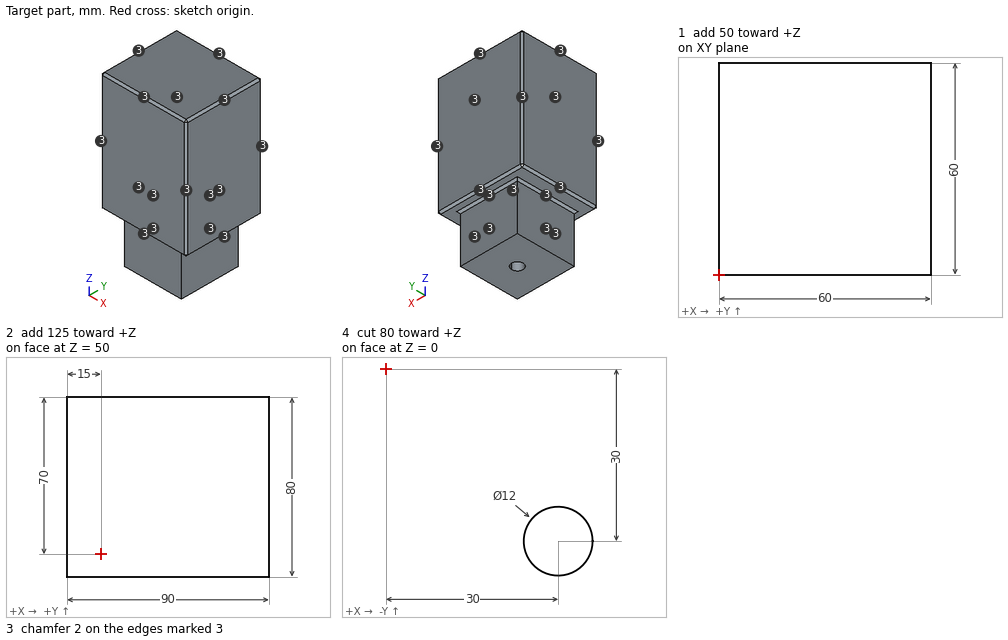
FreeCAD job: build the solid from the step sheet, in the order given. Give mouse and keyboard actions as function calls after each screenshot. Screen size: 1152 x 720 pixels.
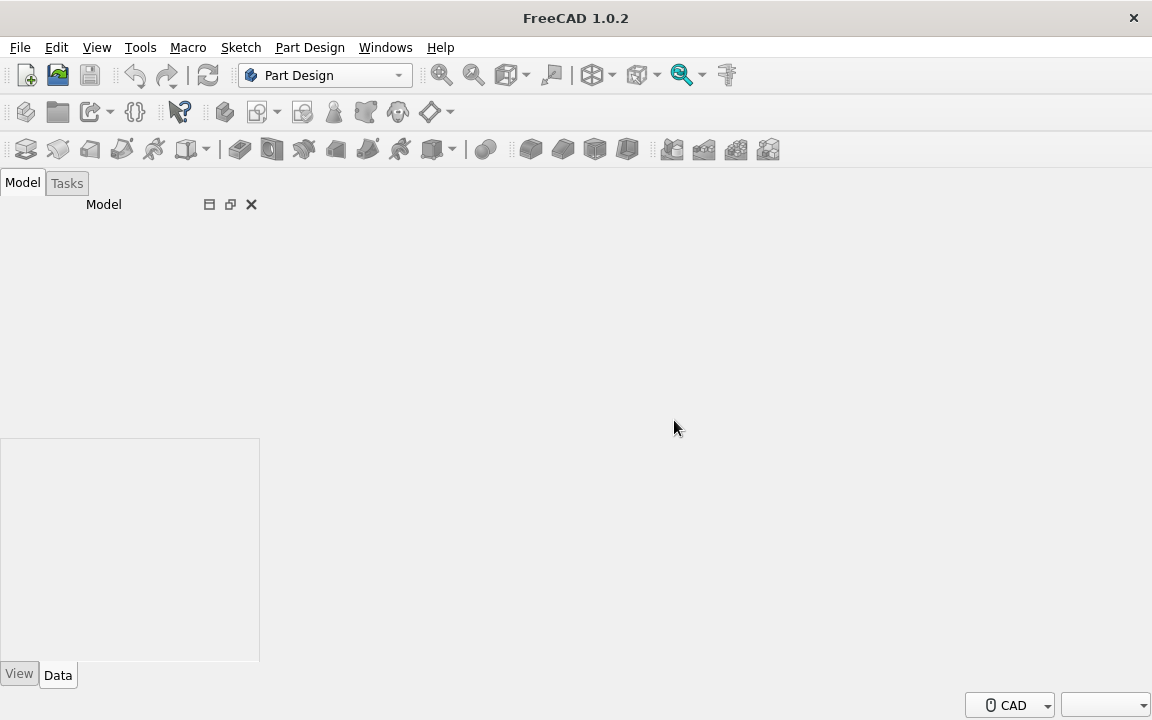
key(ctrl+n)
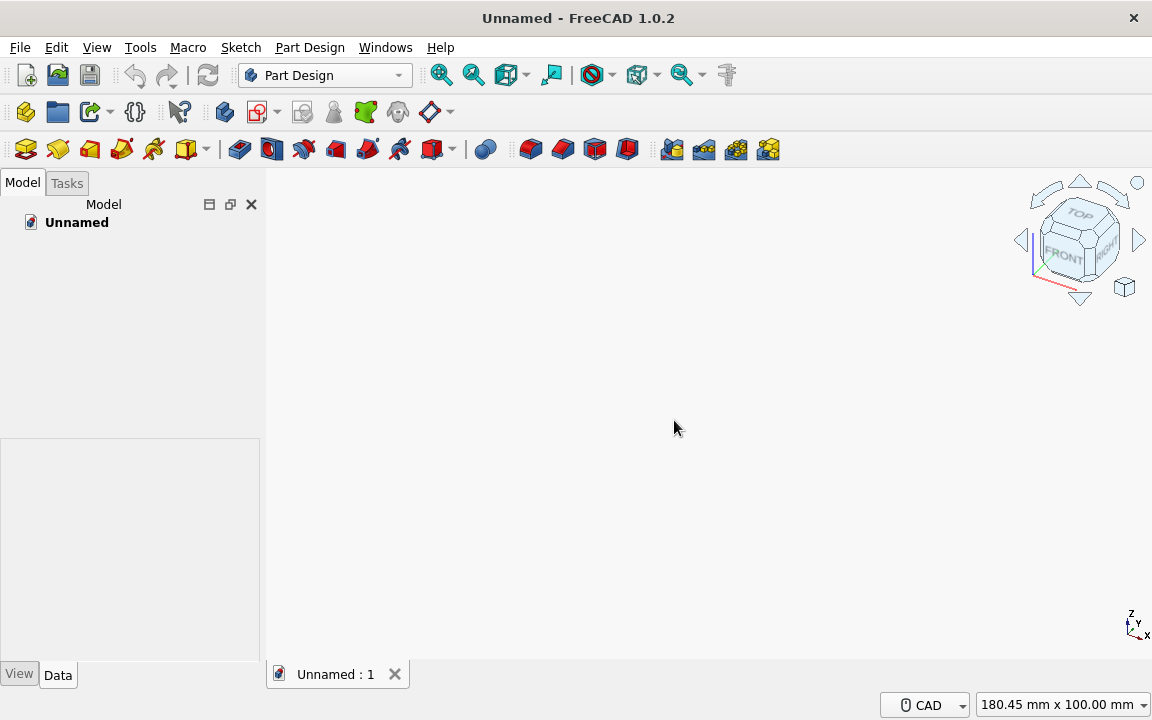
click(258, 112)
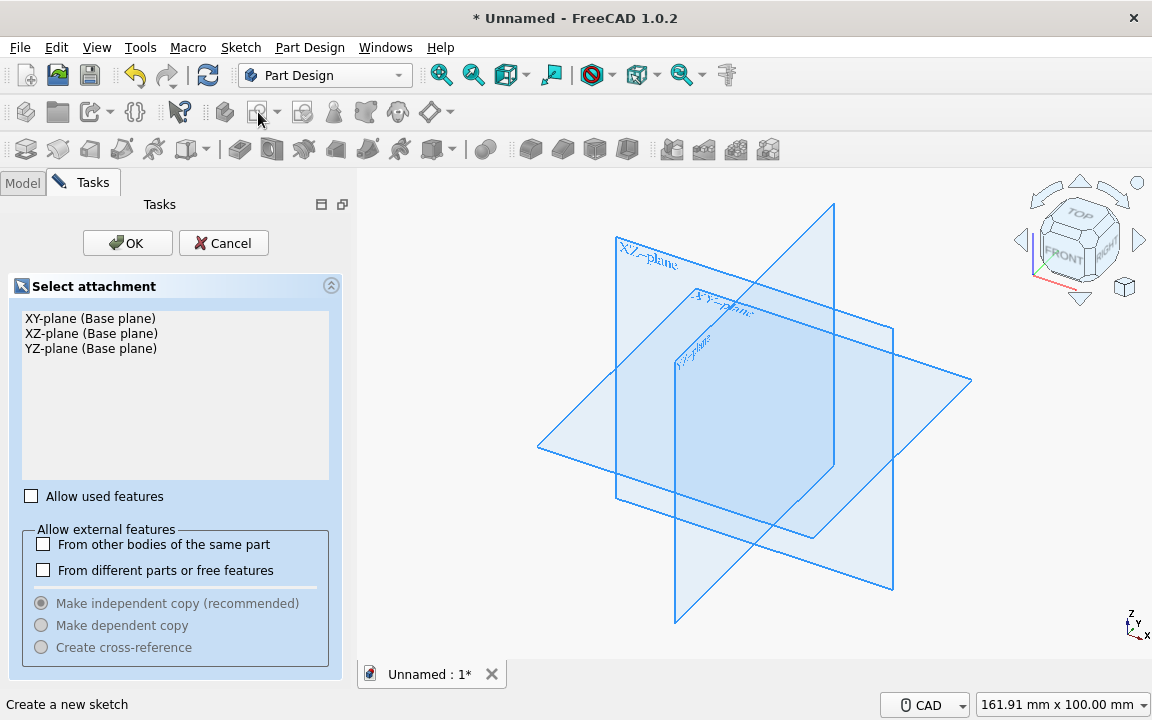
click(82, 318)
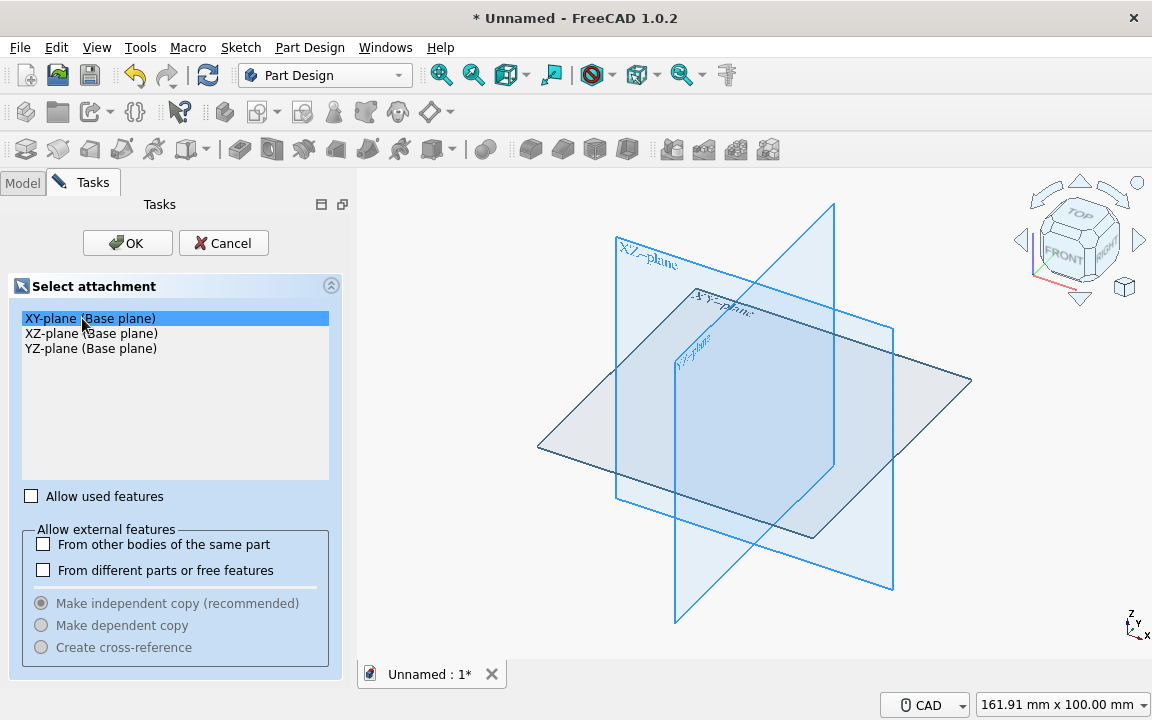
click(128, 243)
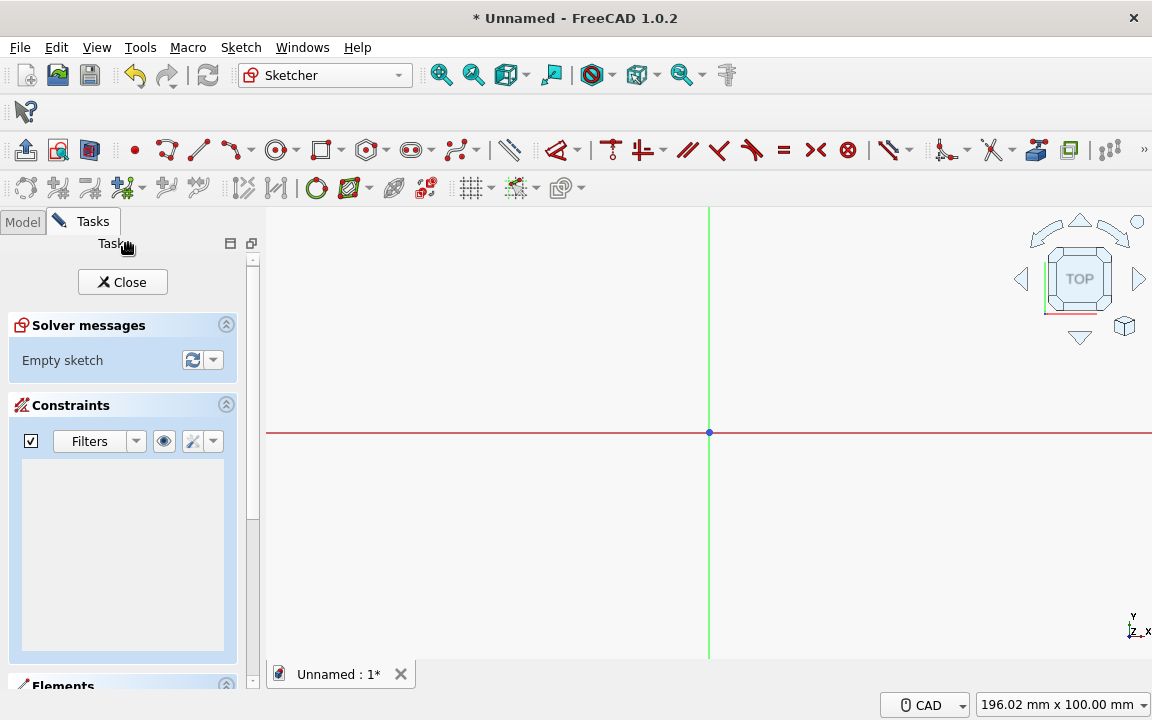
scroll(294, 631, down, 2)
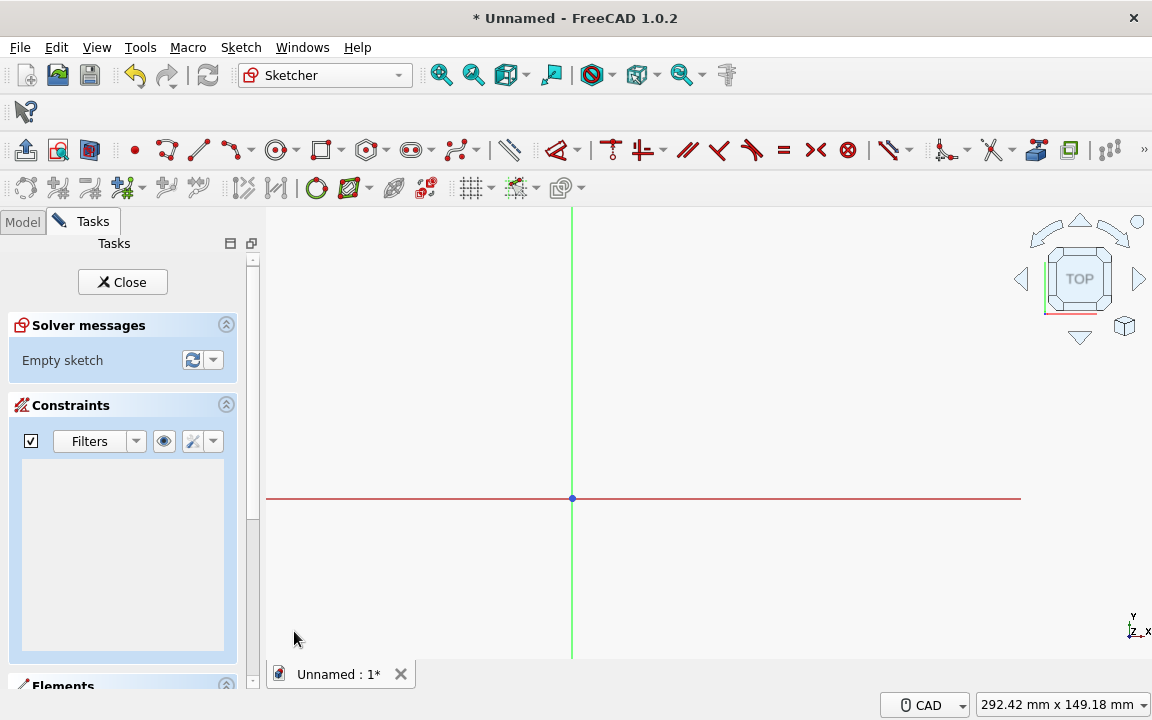
scroll(709, 356, up, 2)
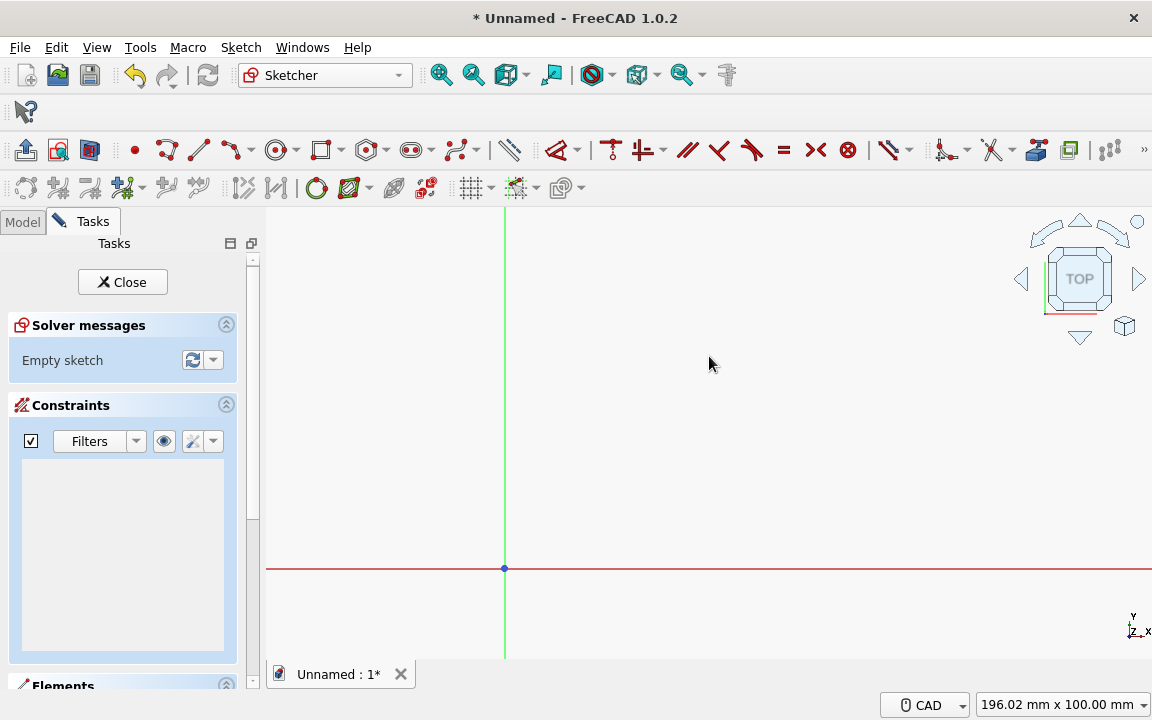
click(322, 150)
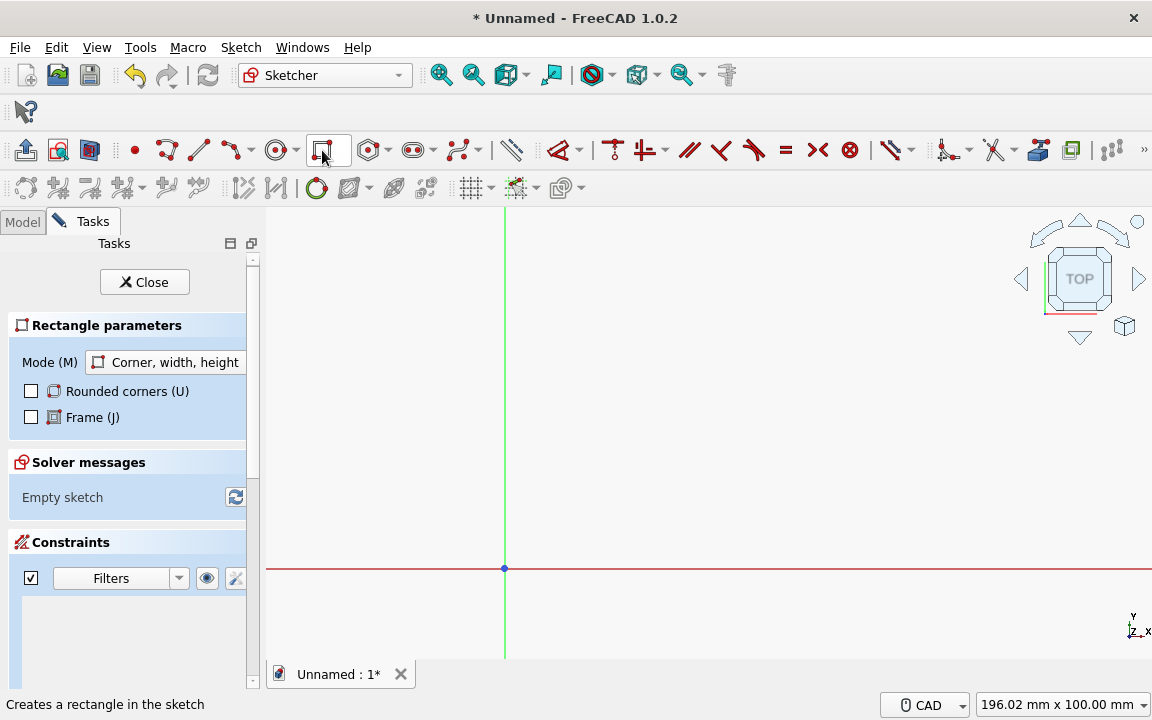
click(505, 569)
move(776, 297)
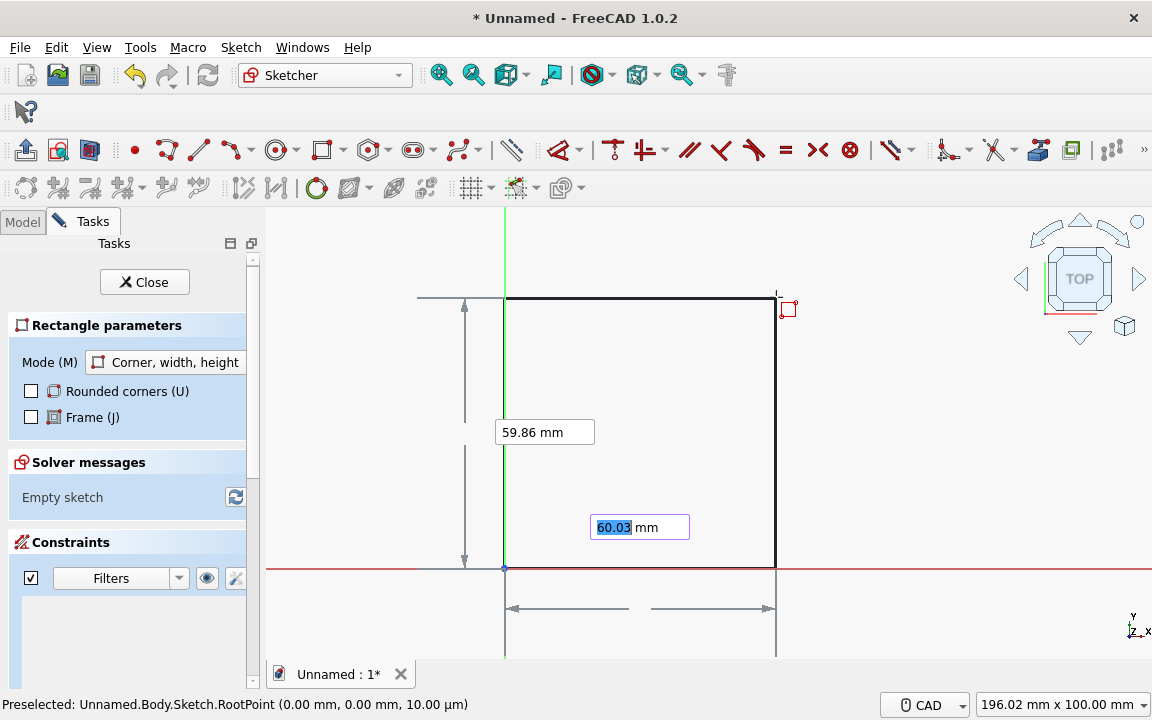
text(60)
key(Tab)
text(60)
key(Return)
key(Escape)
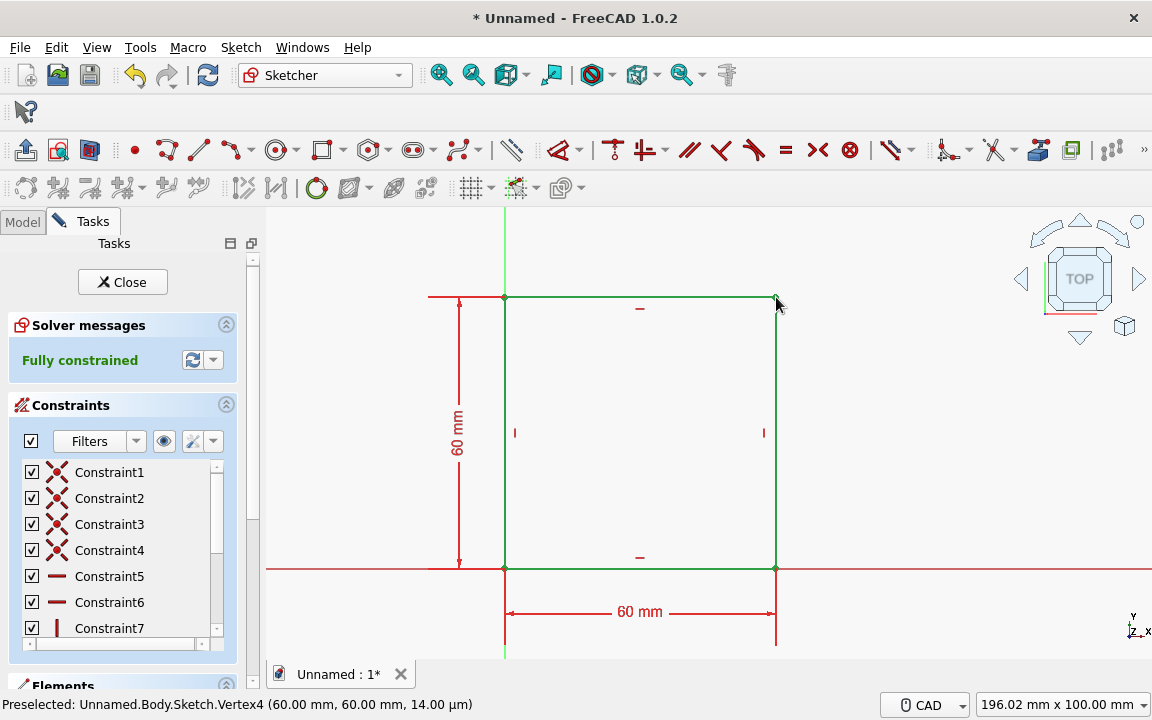
click(123, 282)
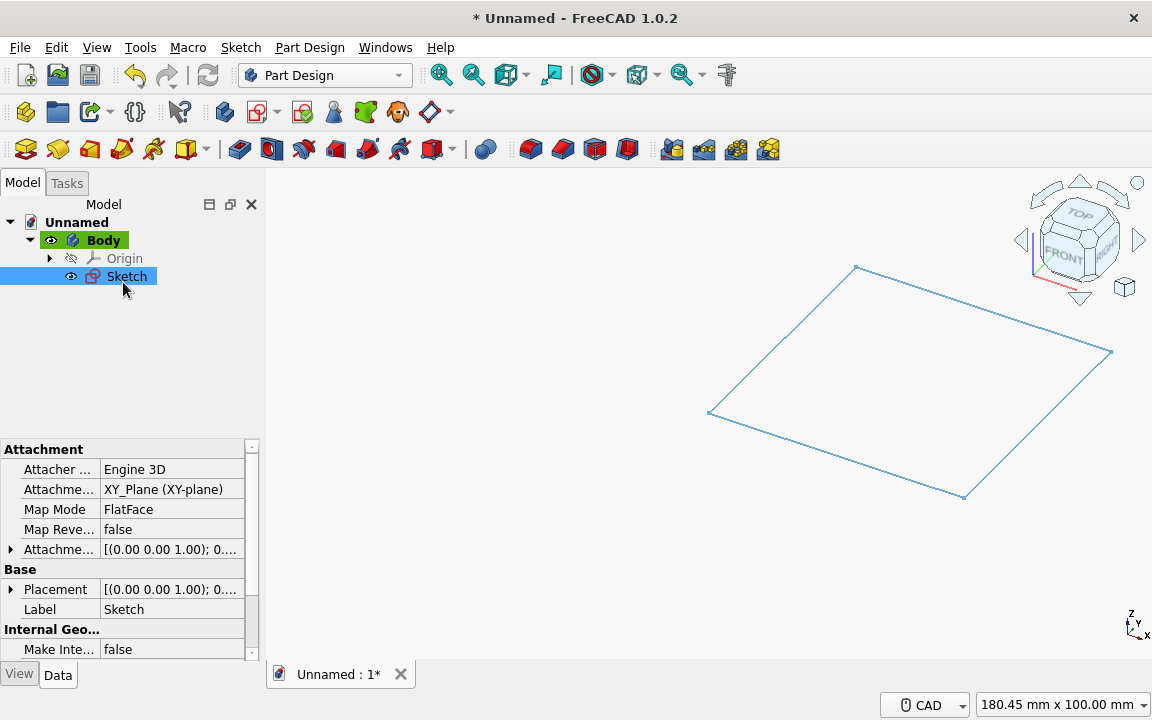
click(26, 150)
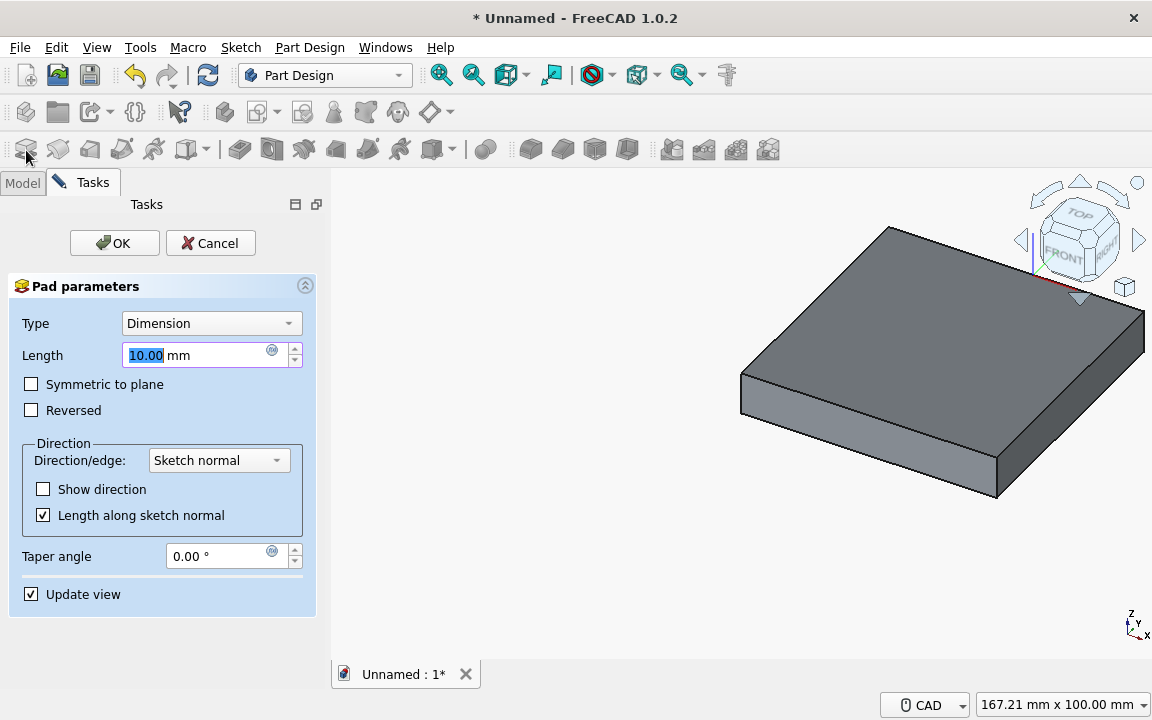
text(50)
key(Tab)